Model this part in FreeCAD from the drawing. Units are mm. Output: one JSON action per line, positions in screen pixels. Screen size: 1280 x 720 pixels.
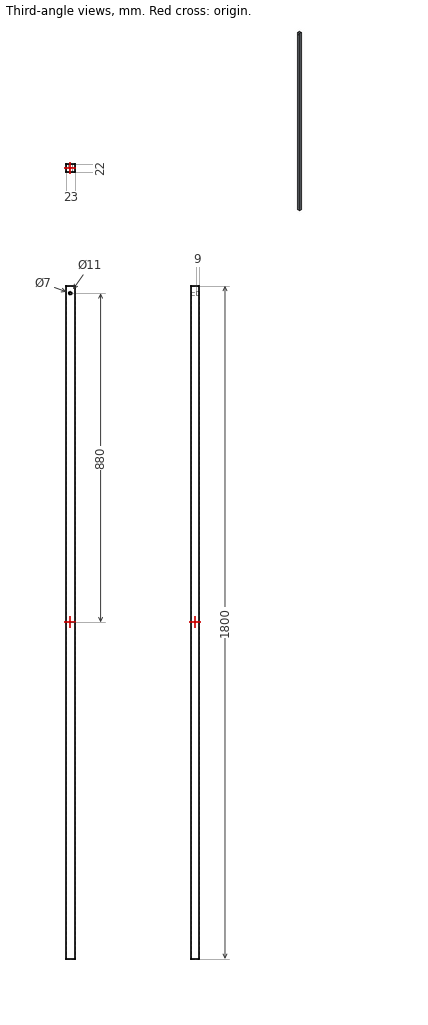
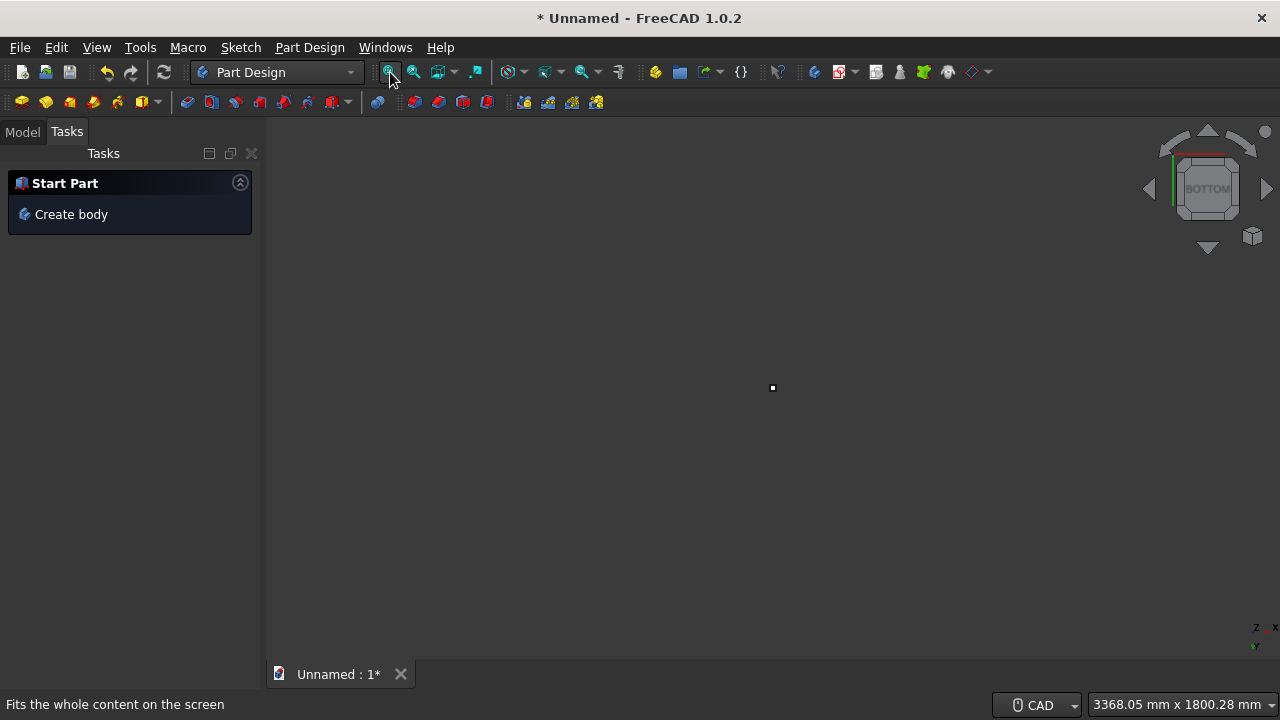
{"action": "key", "text": "4"}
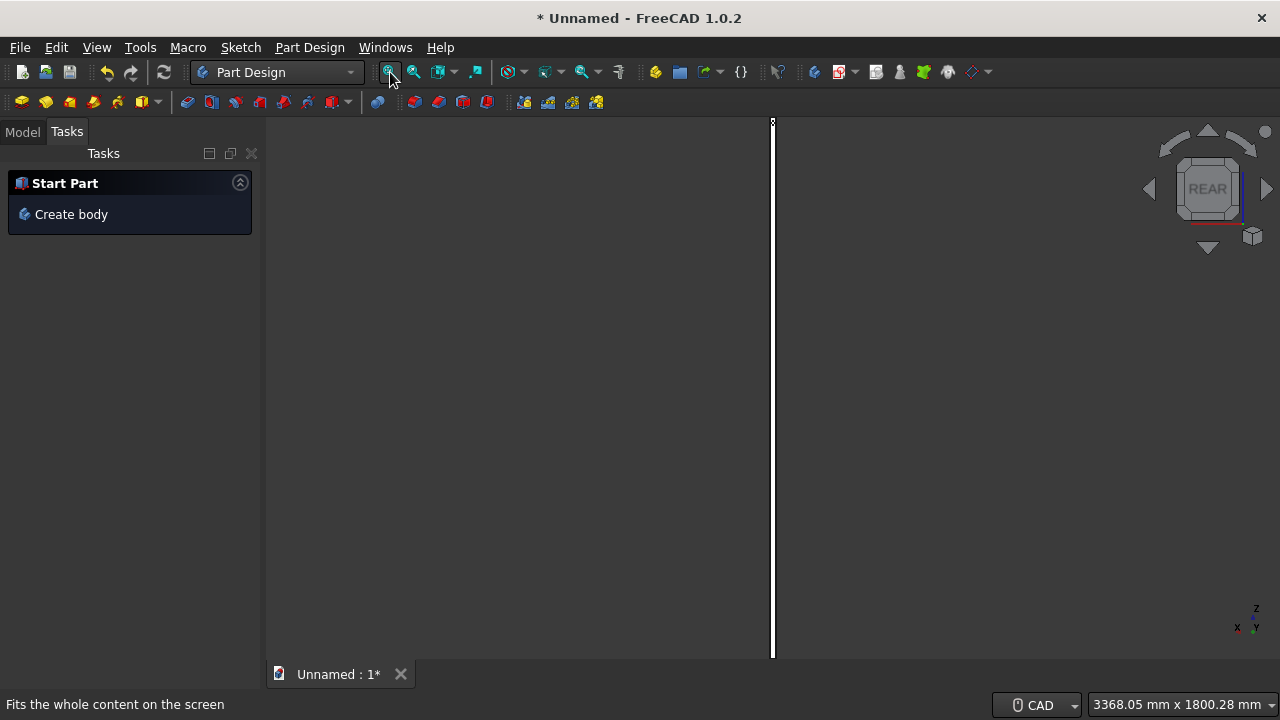
{"action": "left_click", "coordinate": [390, 72]}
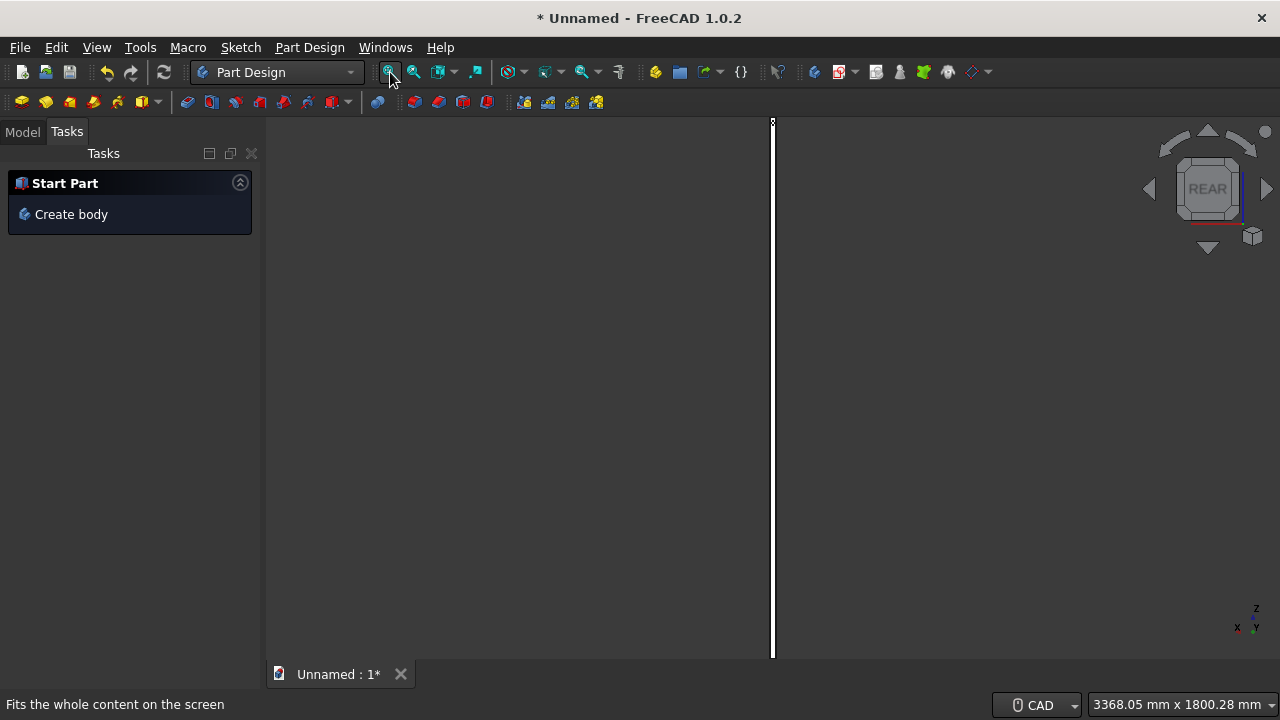
{"action": "key", "text": "3"}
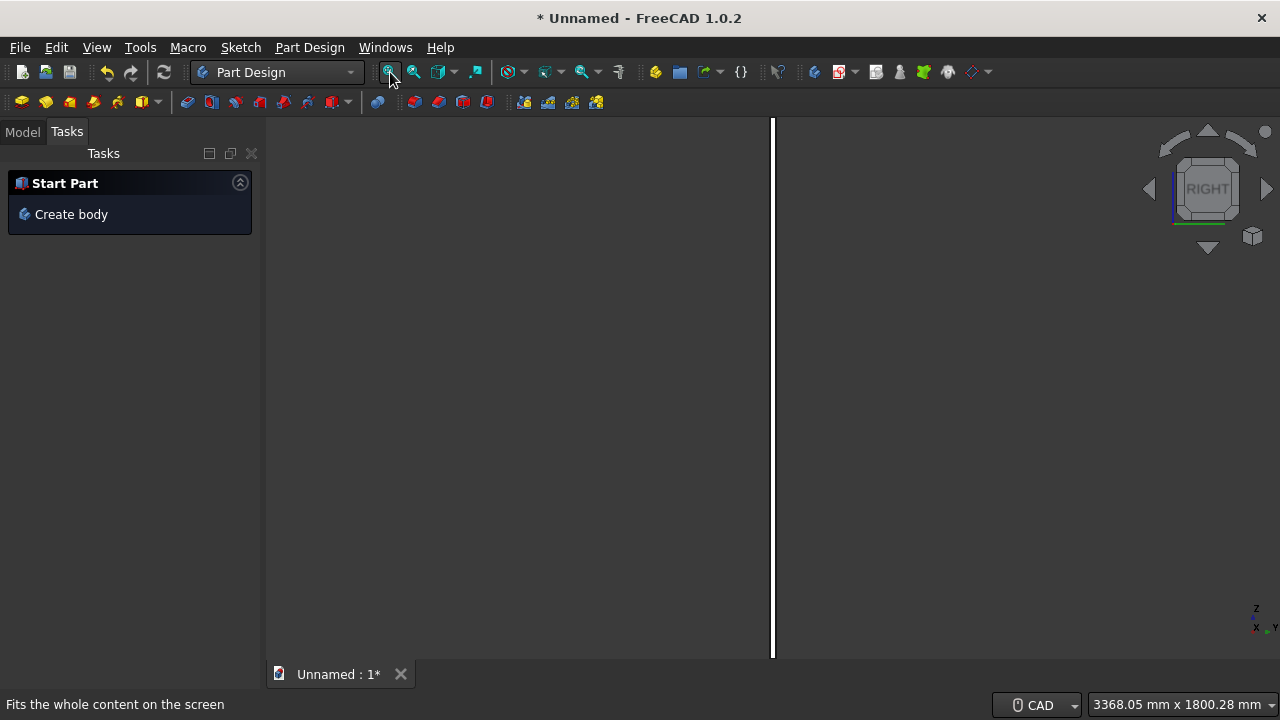
{"action": "left_click", "coordinate": [390, 72]}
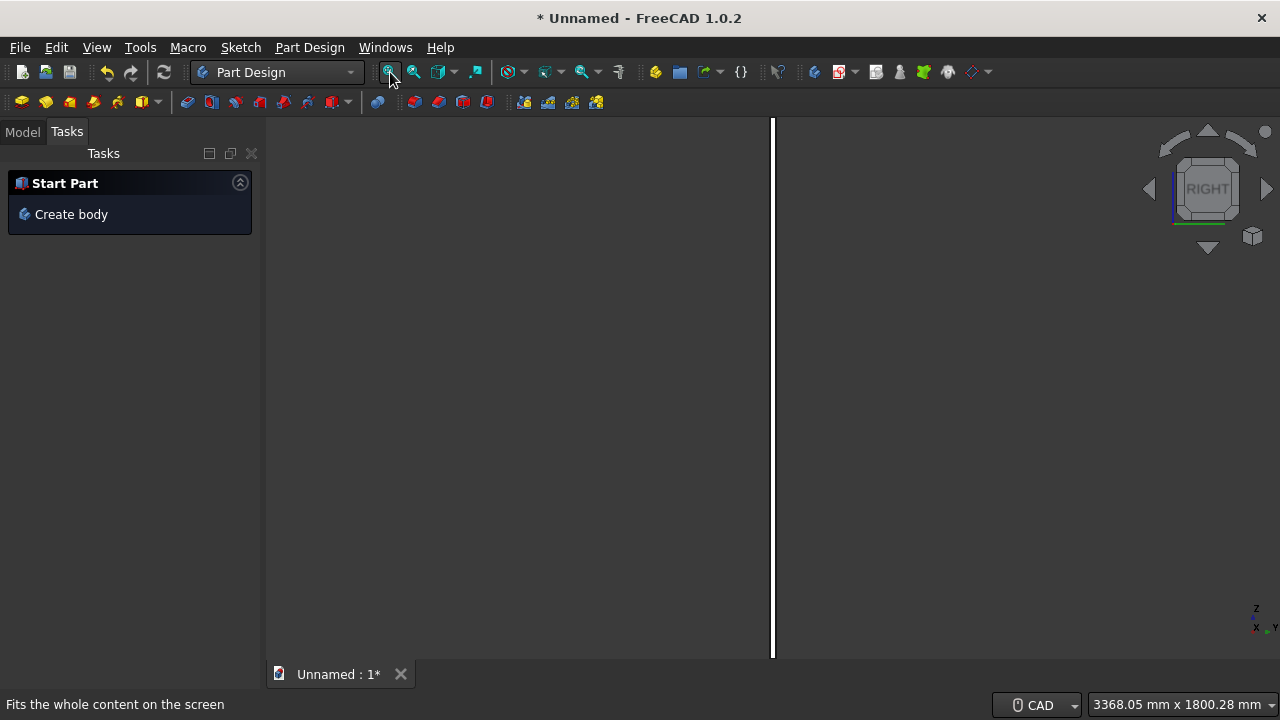
{"action": "left_click", "coordinate": [23, 131]}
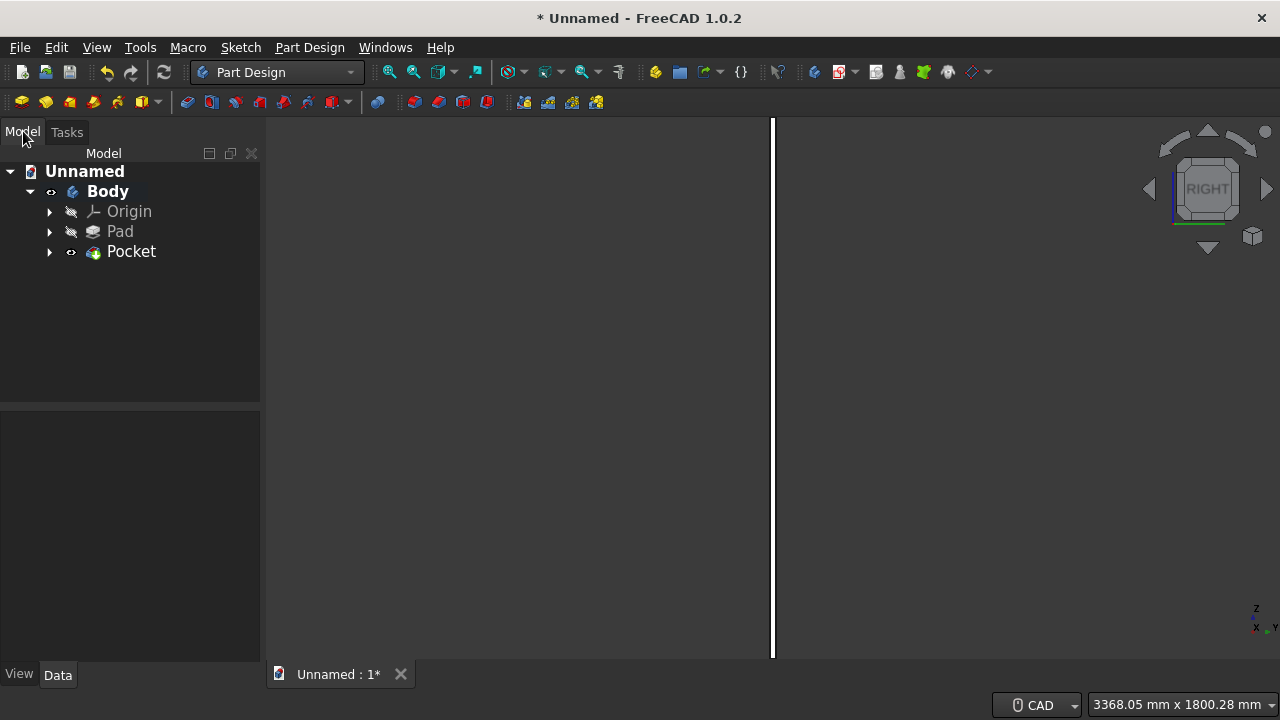
{"action": "left_click", "coordinate": [50, 212]}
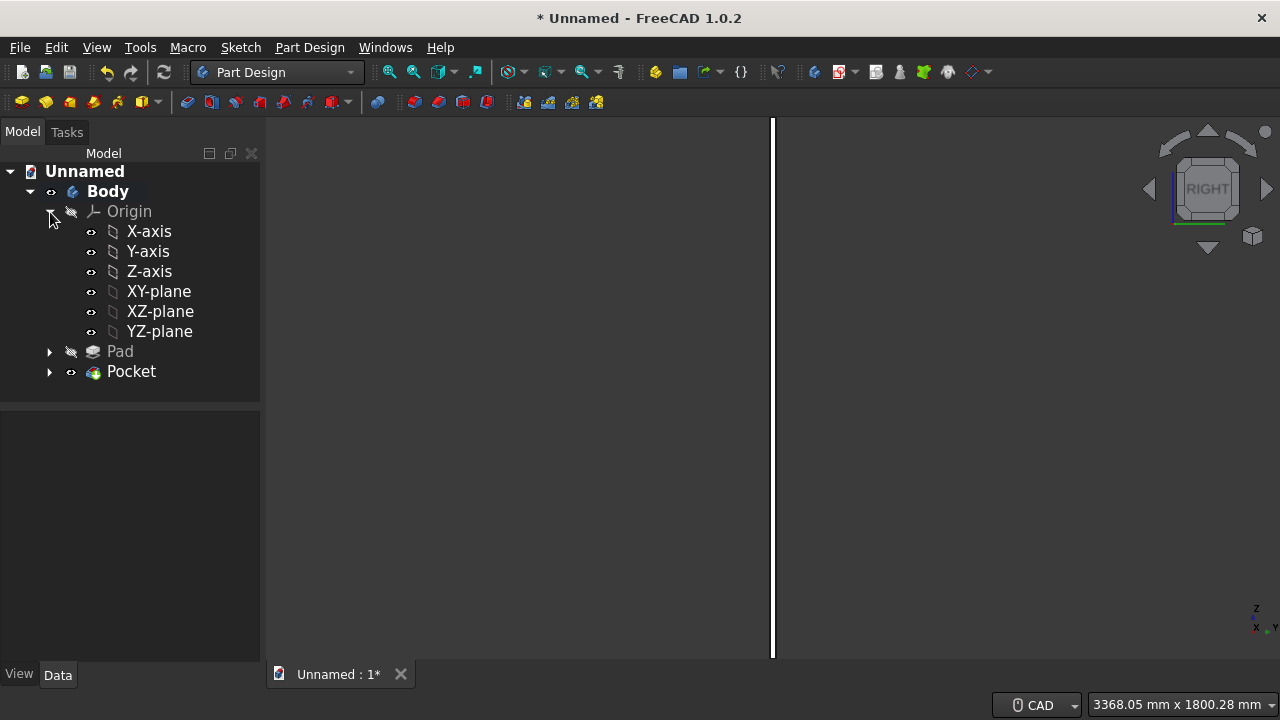
{"action": "left_click", "coordinate": [136, 312]}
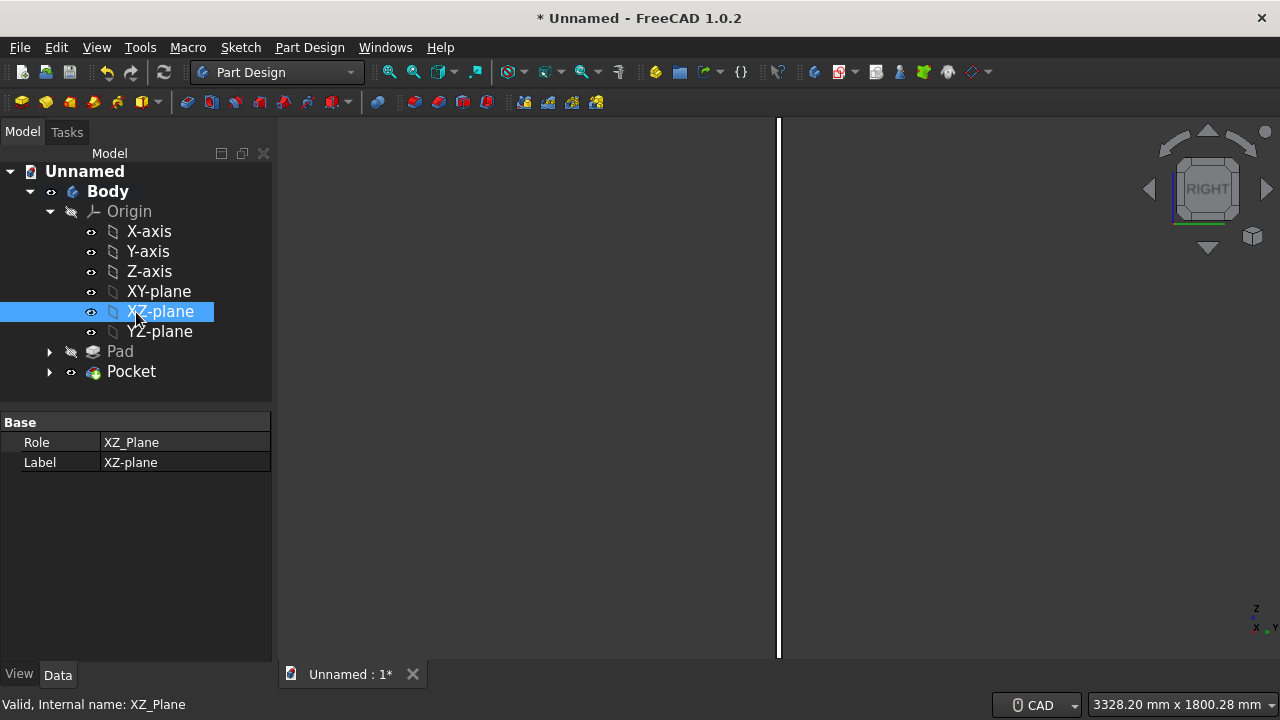
{"action": "left_click", "coordinate": [972, 72]}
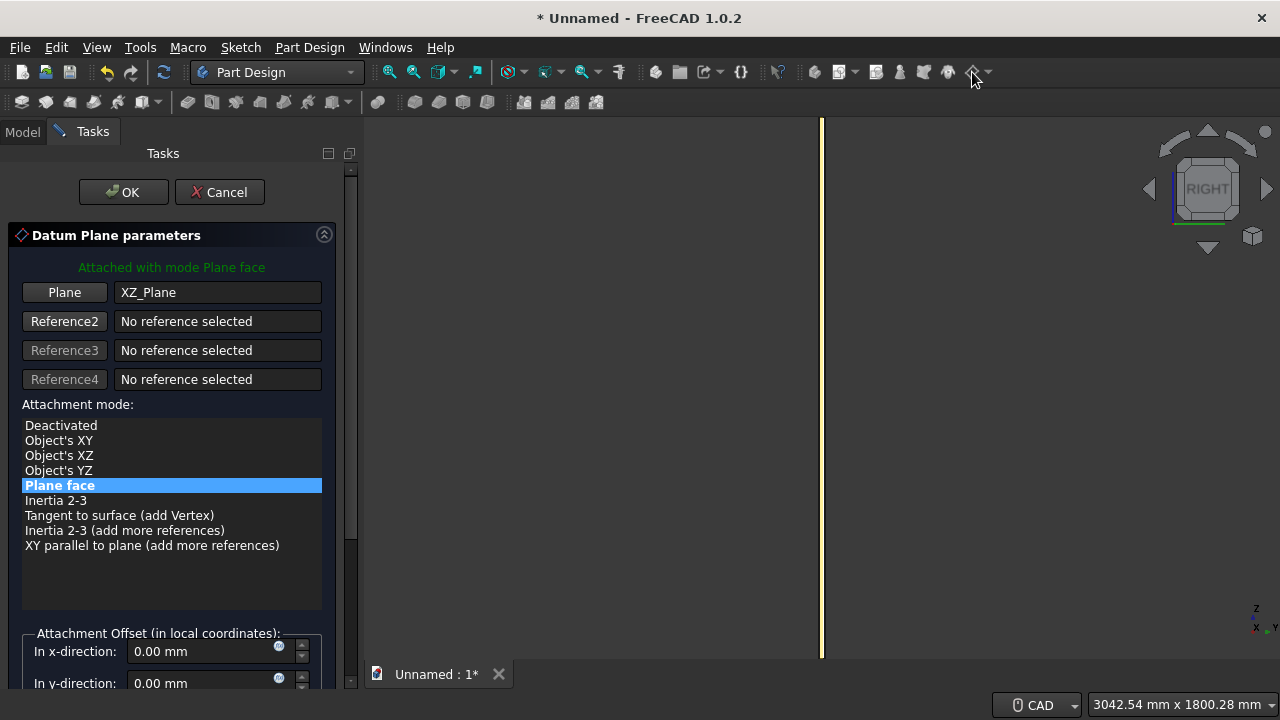
{"action": "scroll", "coordinate": [351, 426], "scroll_direction": "down", "scroll_amount": 2}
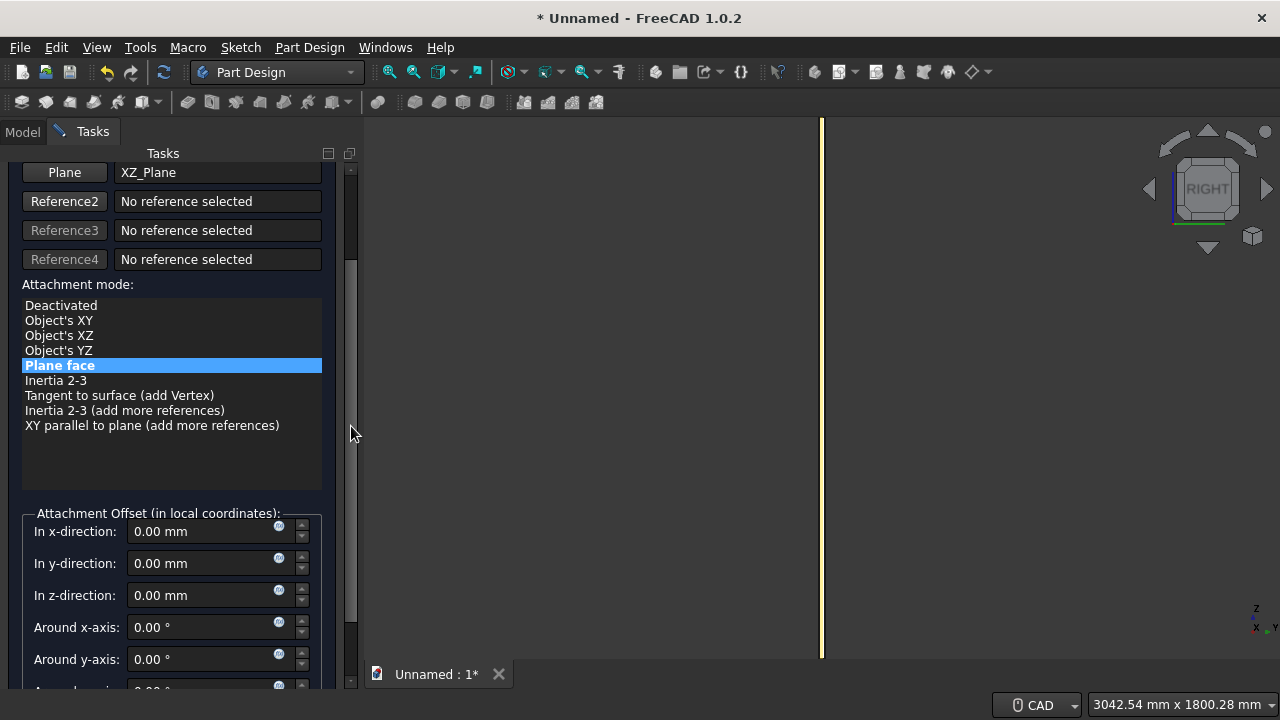
{"action": "triple_click", "coordinate": [210, 595]}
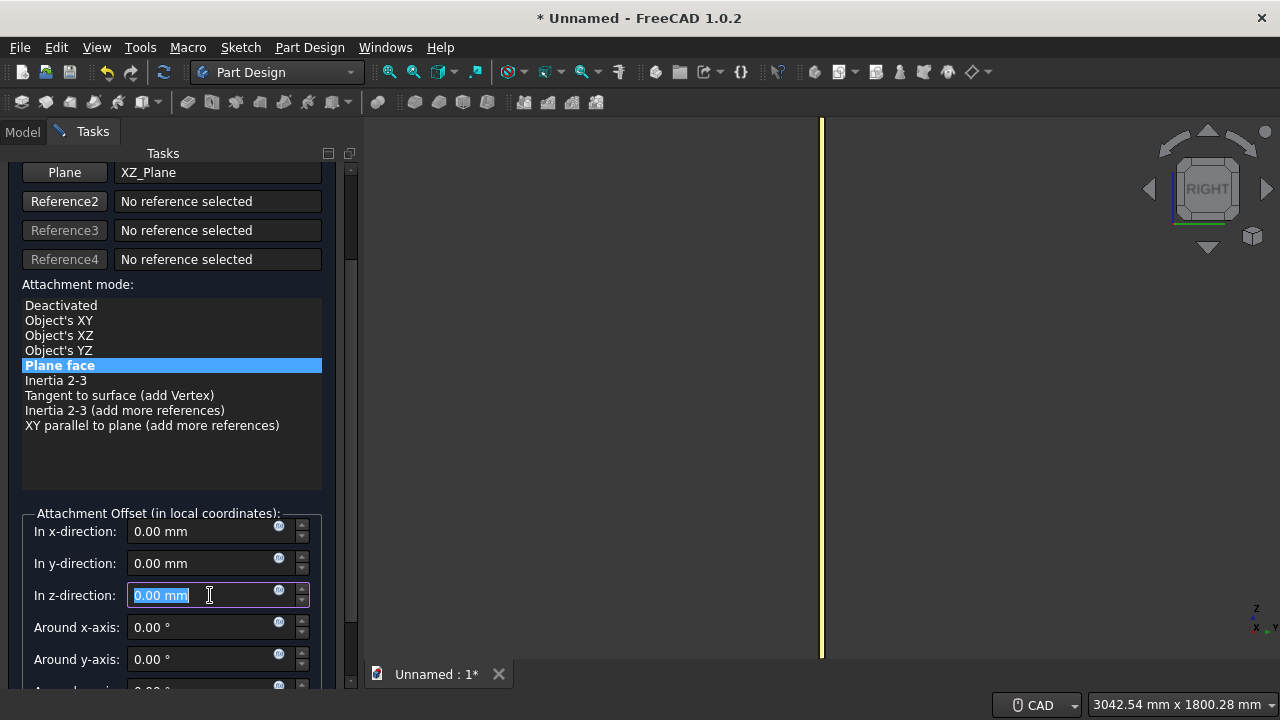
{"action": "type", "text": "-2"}
{"action": "key", "text": "Tab"}